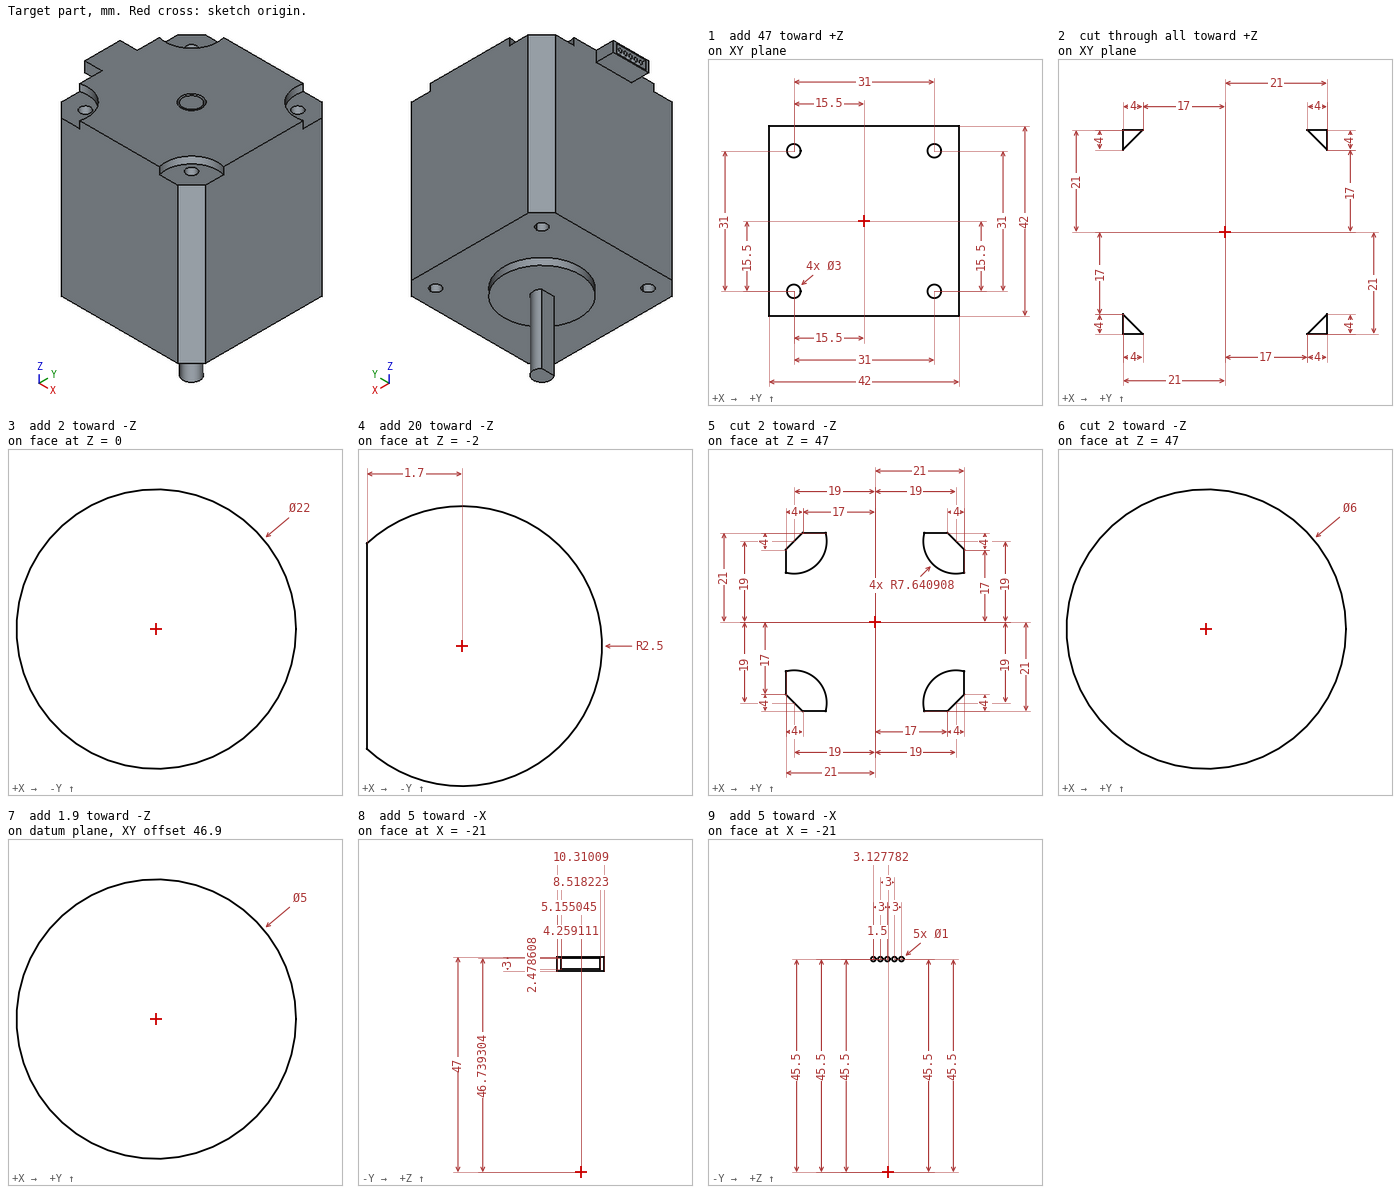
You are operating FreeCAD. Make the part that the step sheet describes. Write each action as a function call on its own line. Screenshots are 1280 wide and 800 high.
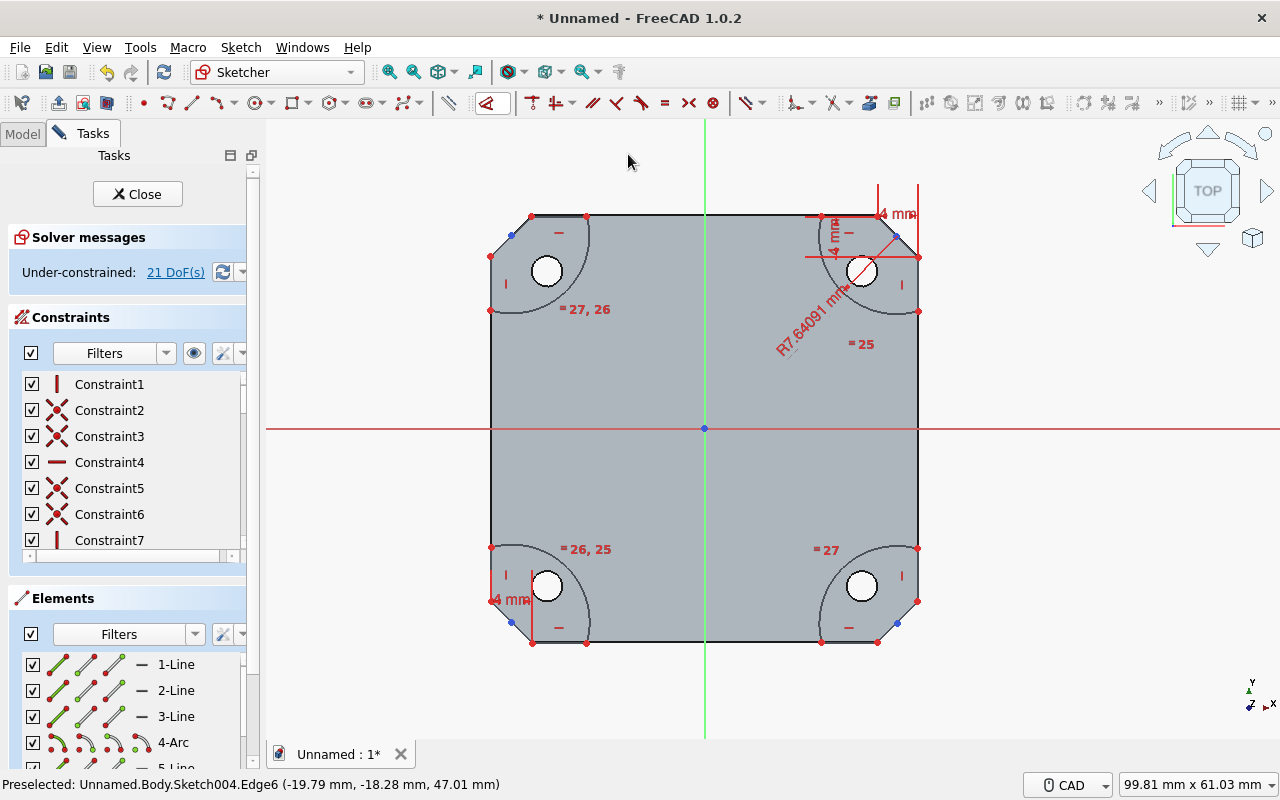
click(504, 614)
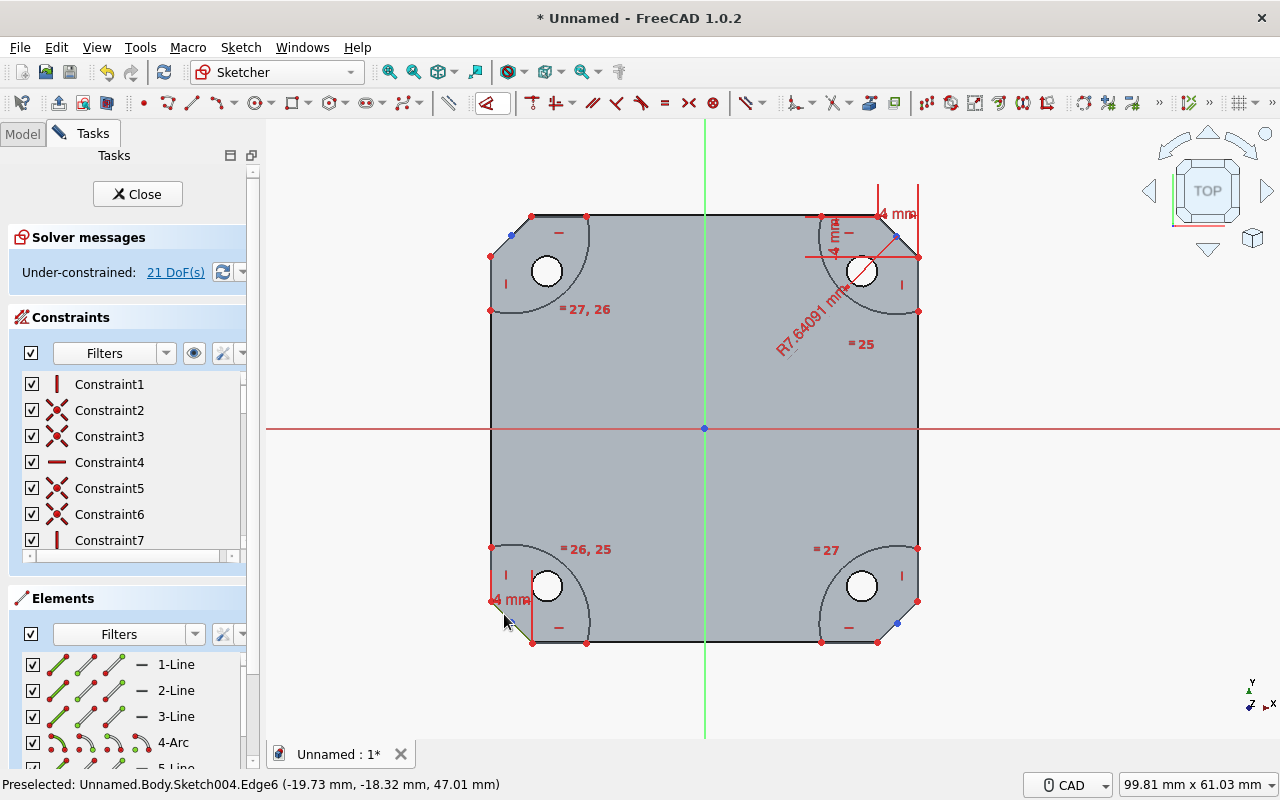
click(504, 104)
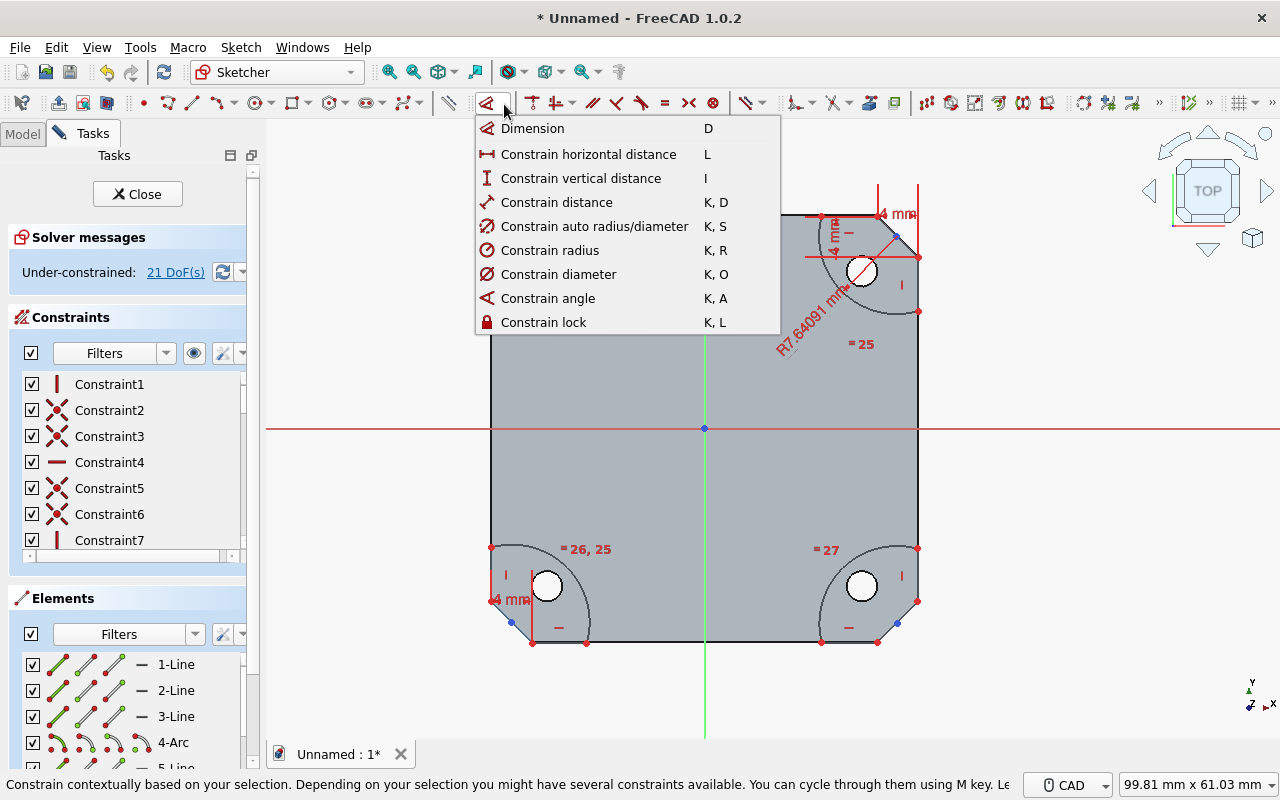
click(628, 178)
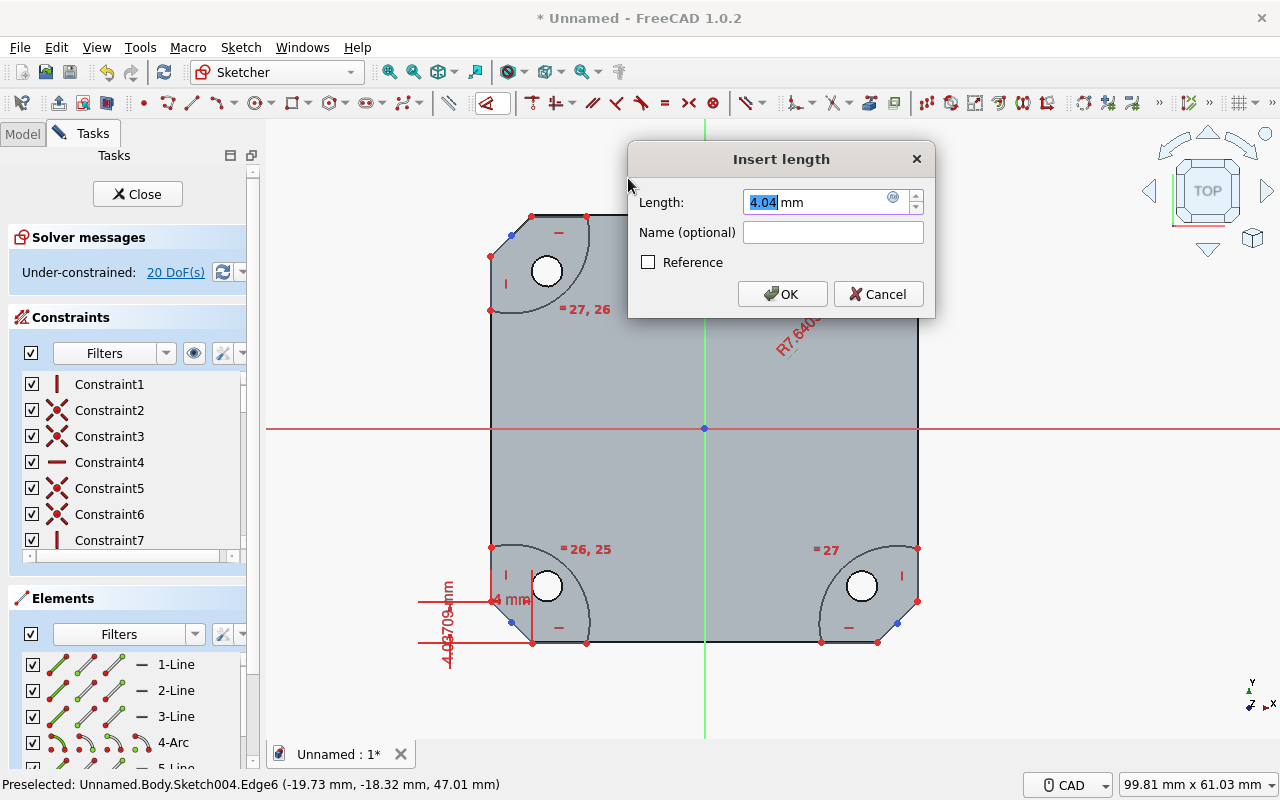
text(4)
key(Return)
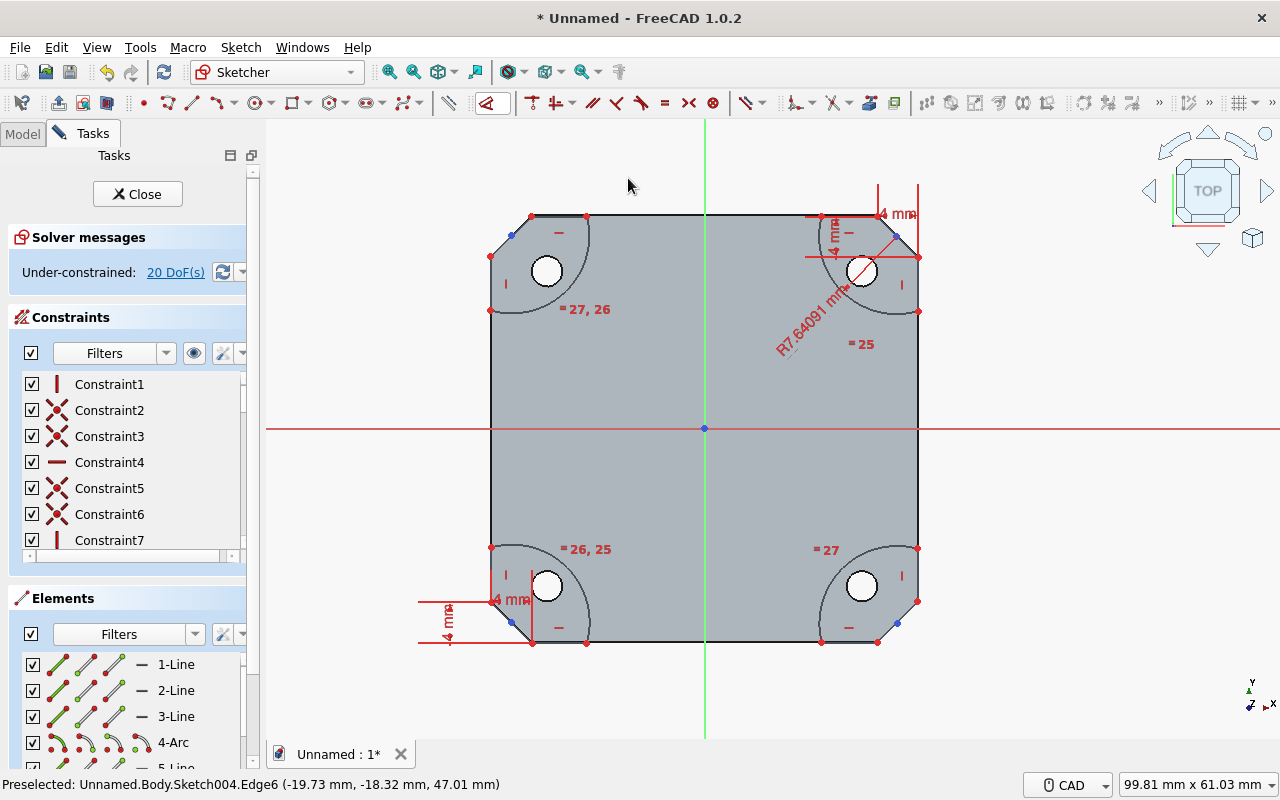
click(520, 229)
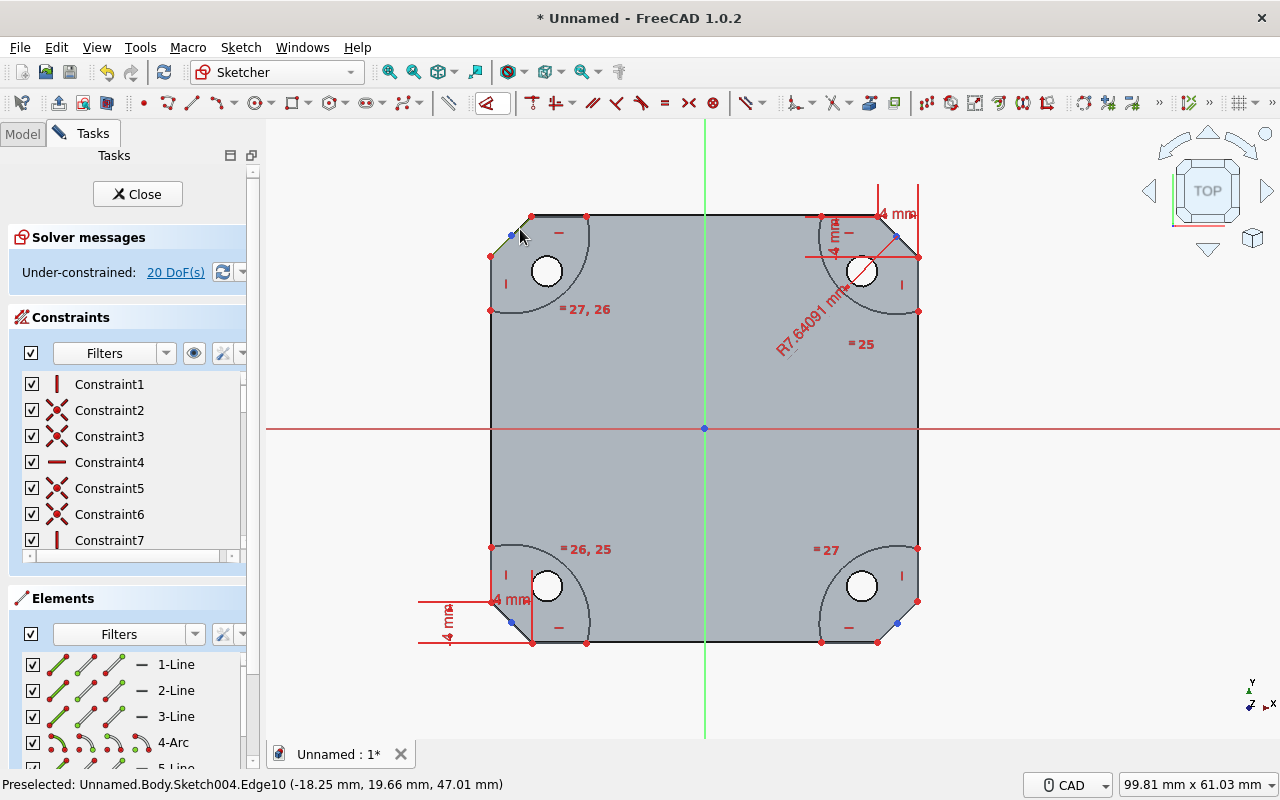
key(l)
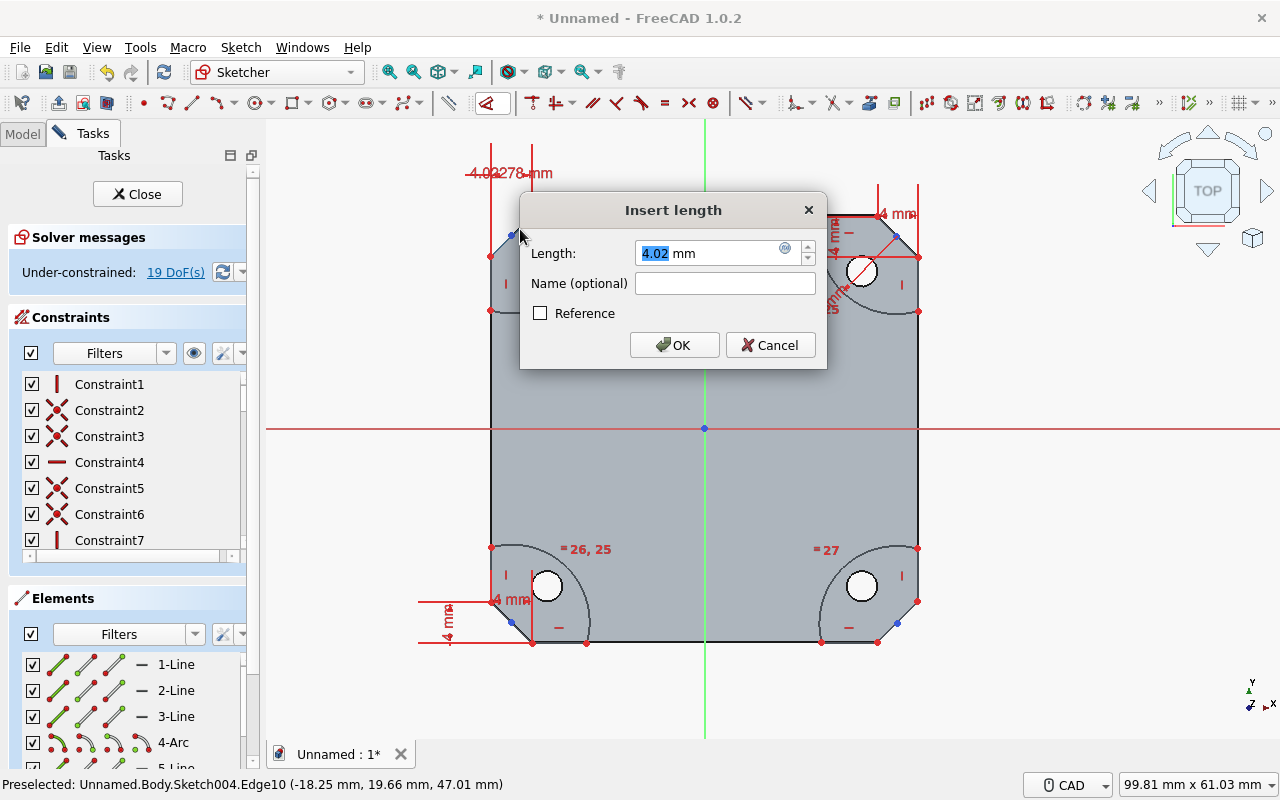
text(4)
key(Return)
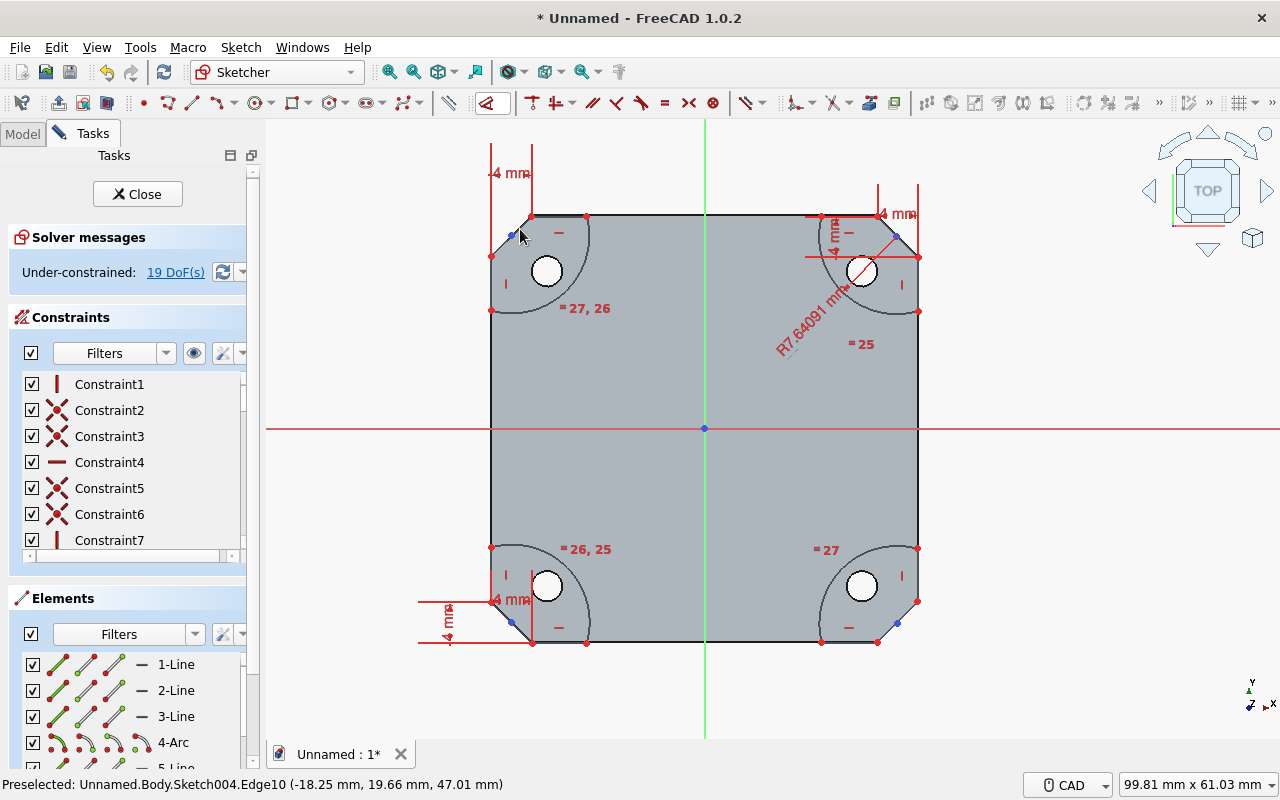
click(520, 229)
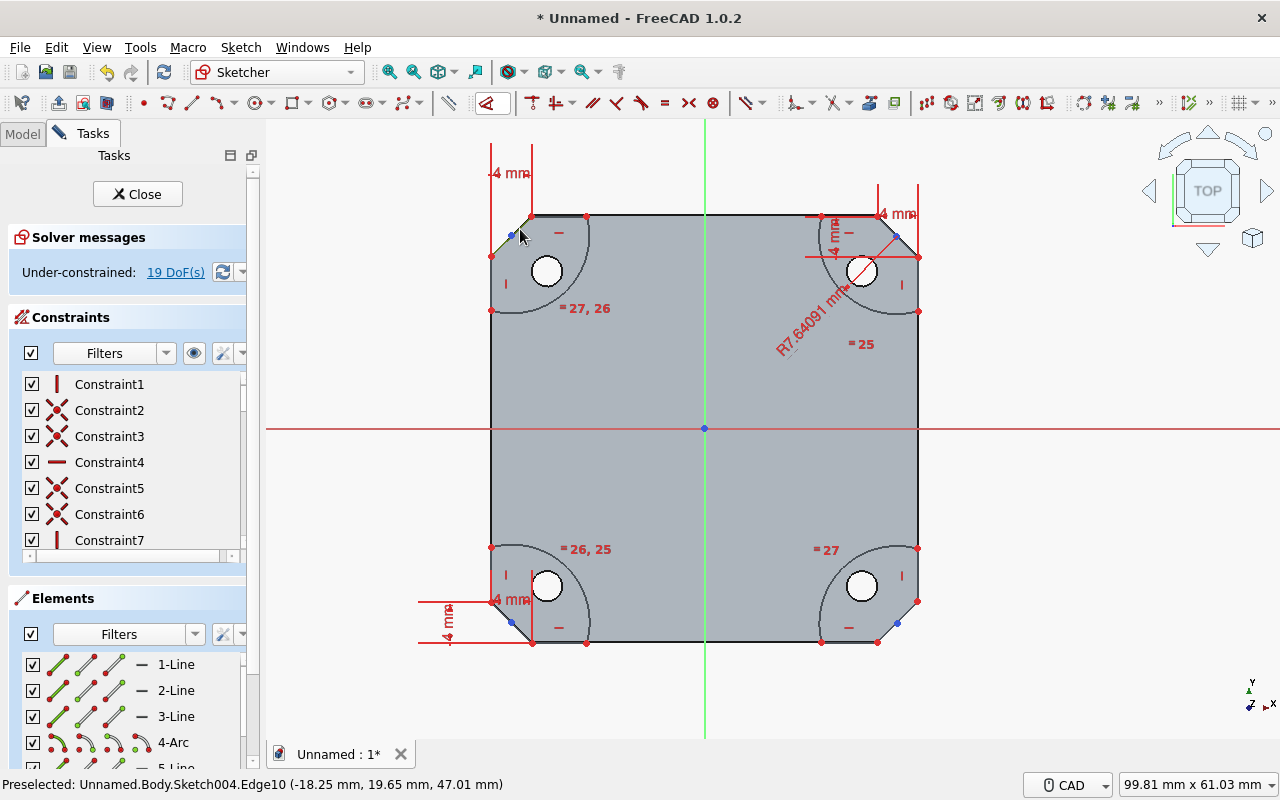
key(i)